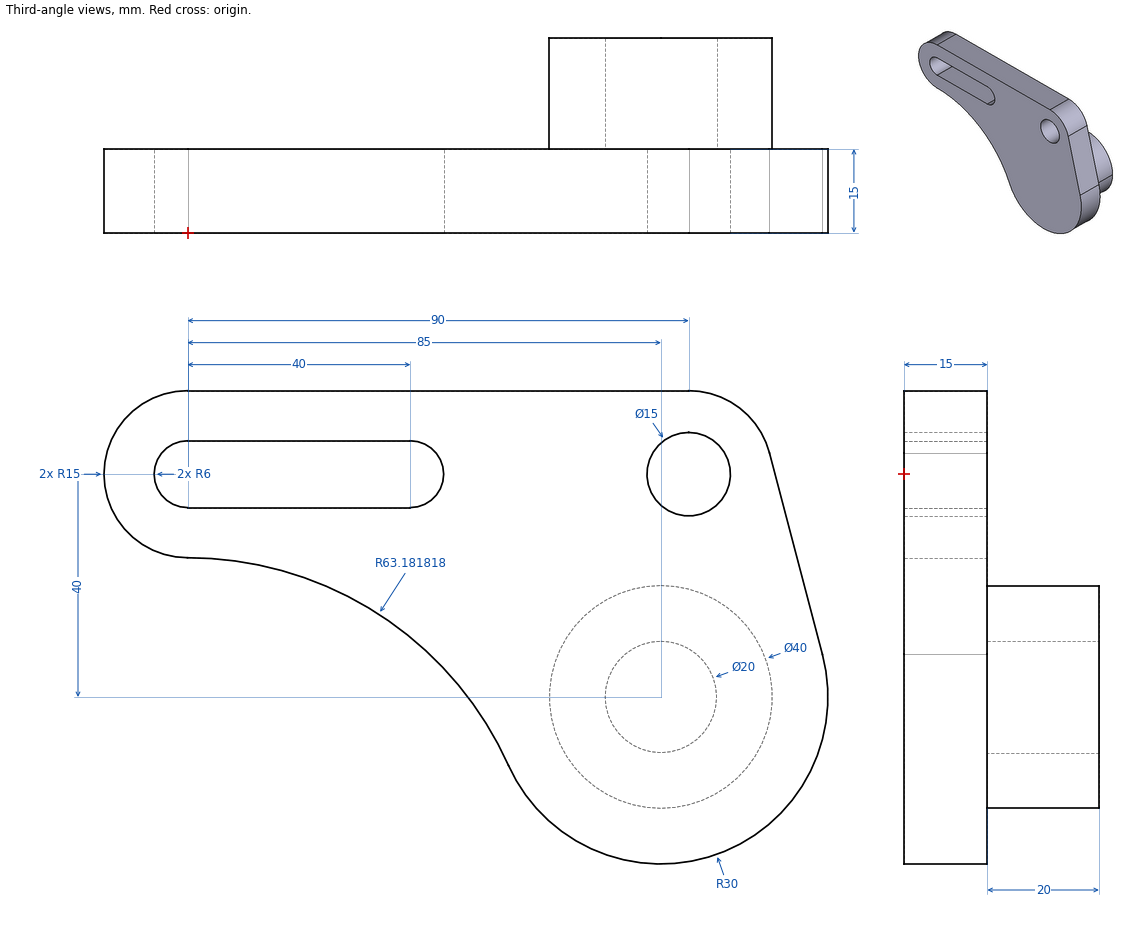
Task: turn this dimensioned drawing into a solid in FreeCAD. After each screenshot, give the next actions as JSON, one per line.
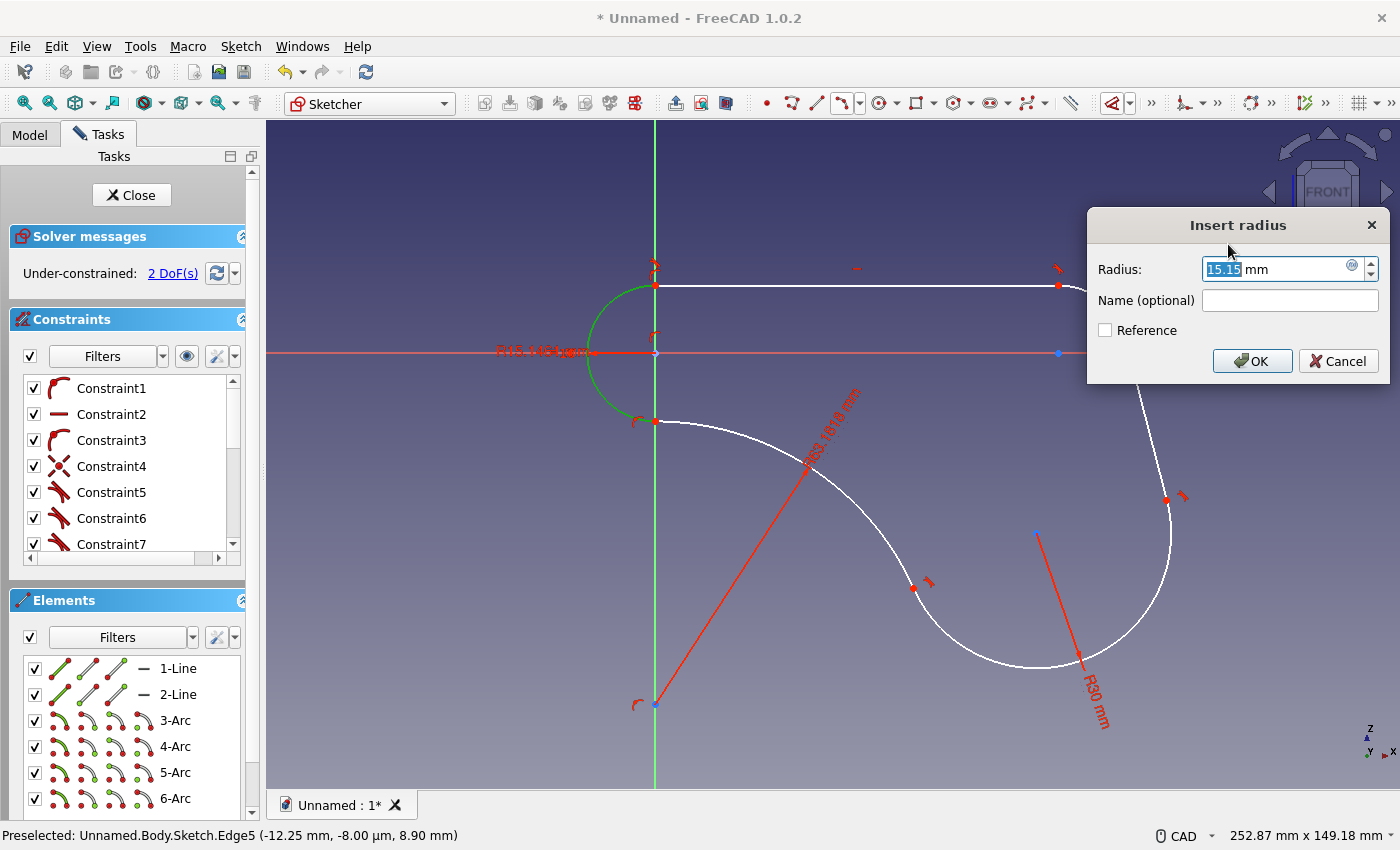
{"action": "type", "text": "15"}
{"action": "key", "text": "Return"}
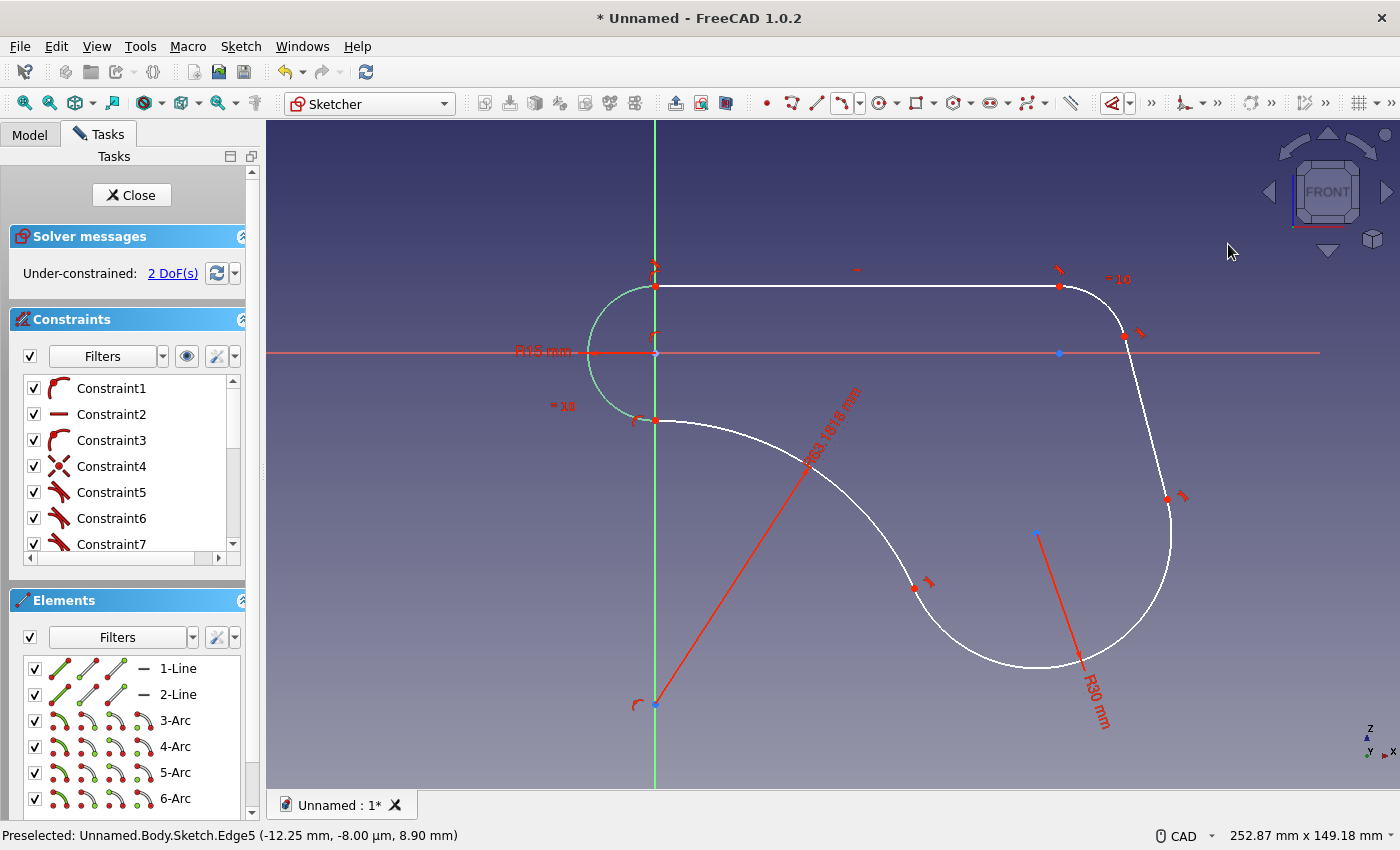
{"action": "left_click", "coordinate": [777, 286]}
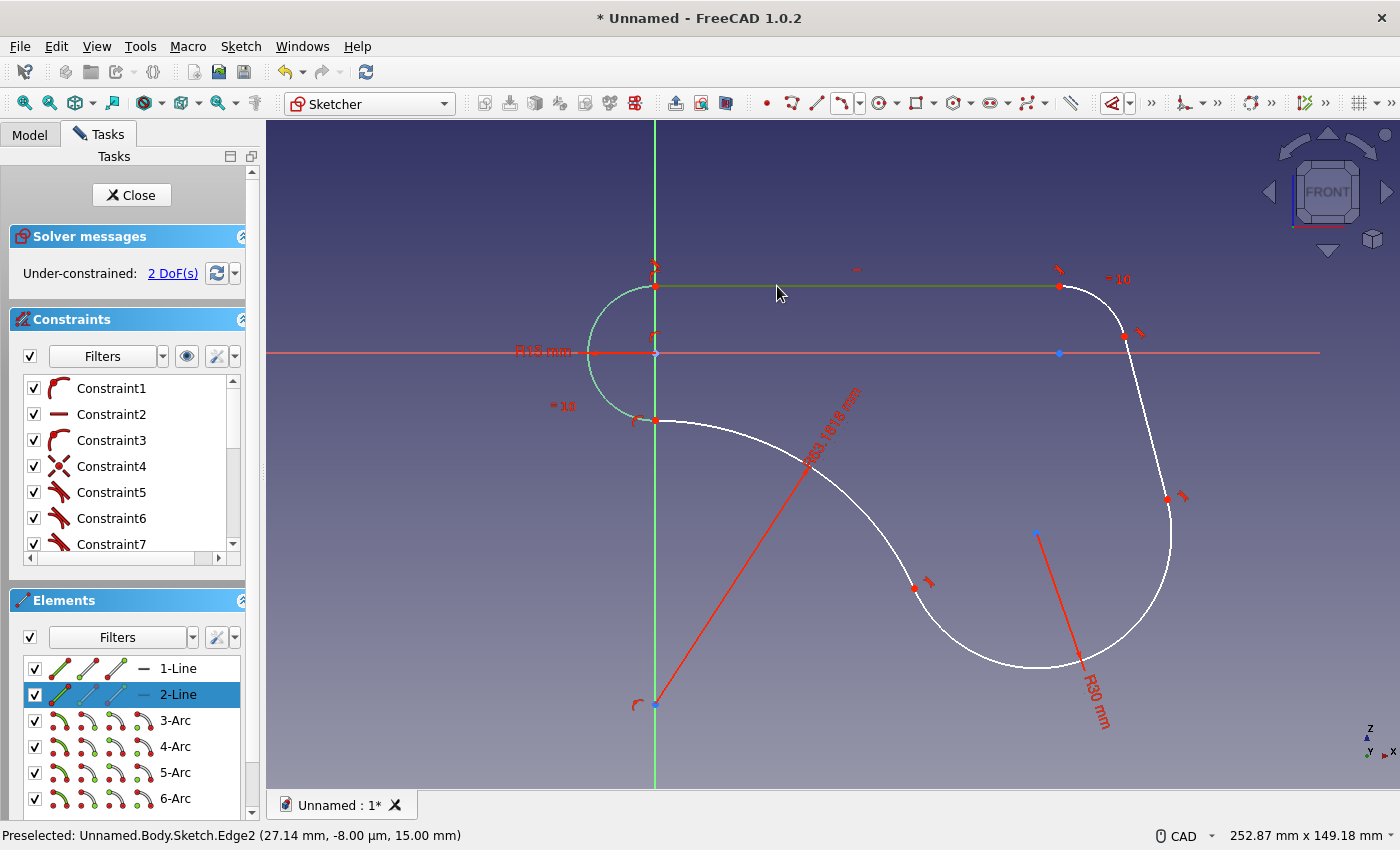
{"action": "left_click", "coordinate": [1130, 104]}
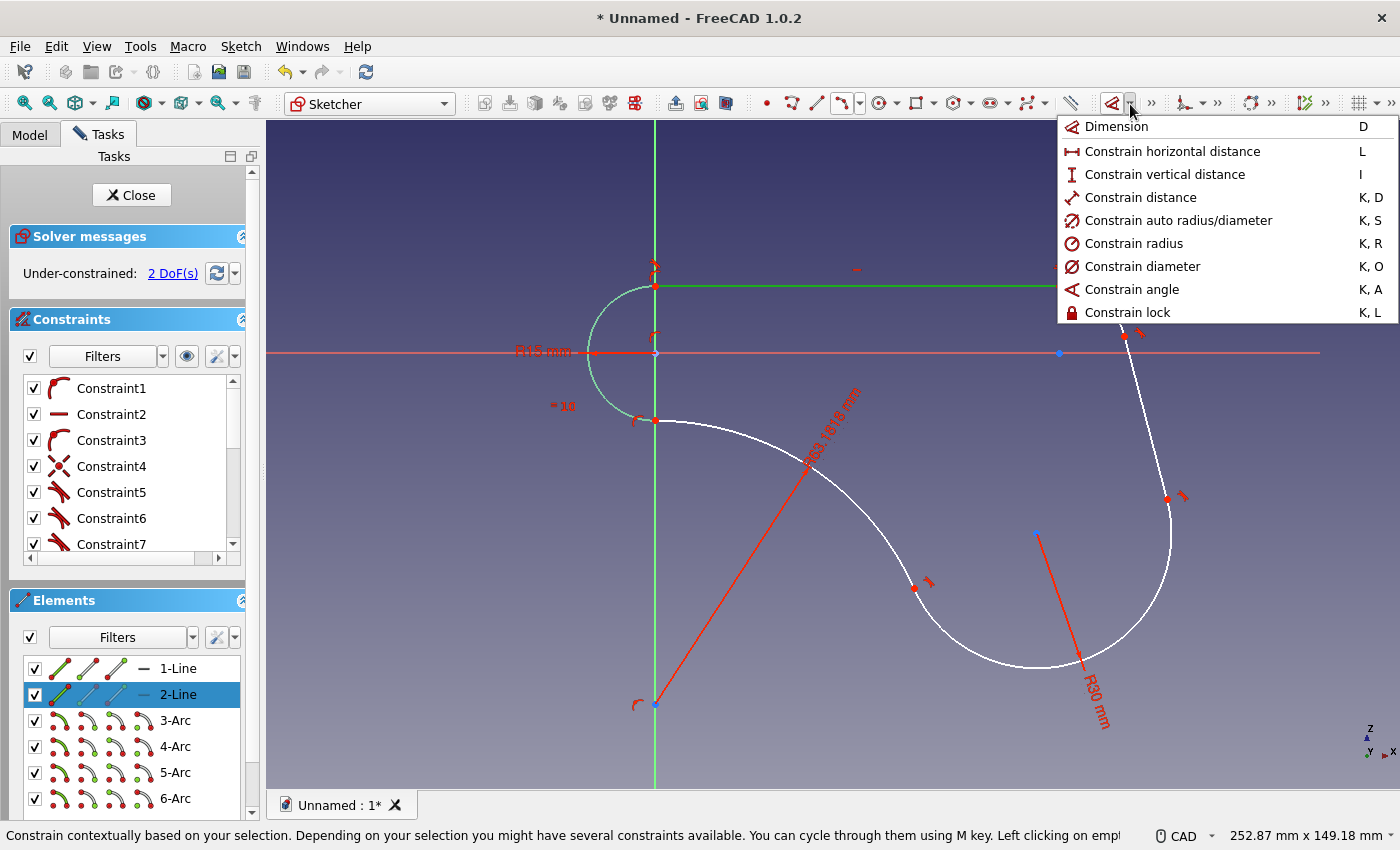
{"action": "left_click", "coordinate": [1228, 152]}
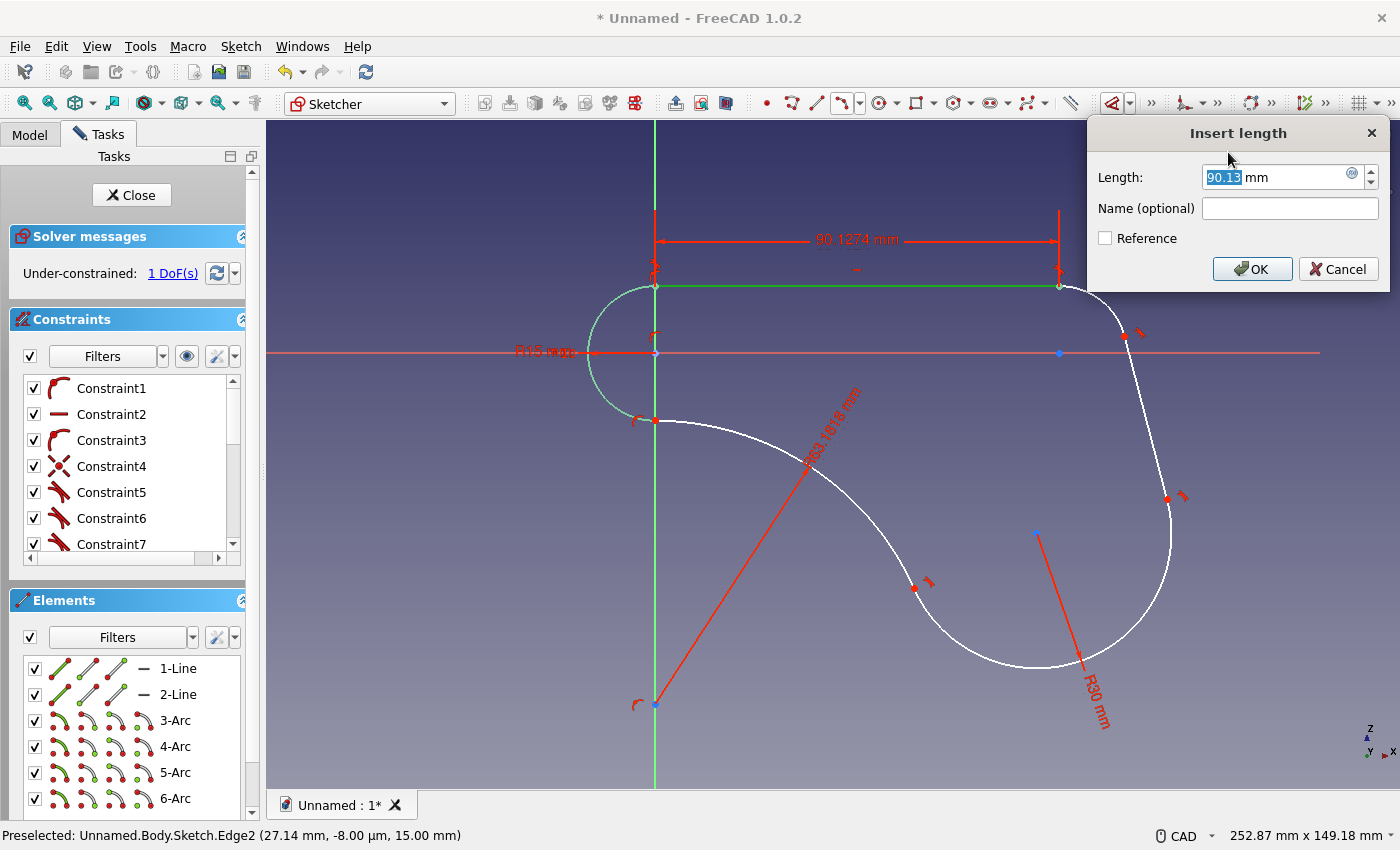
{"action": "type", "text": "90"}
{"action": "key", "text": "Return"}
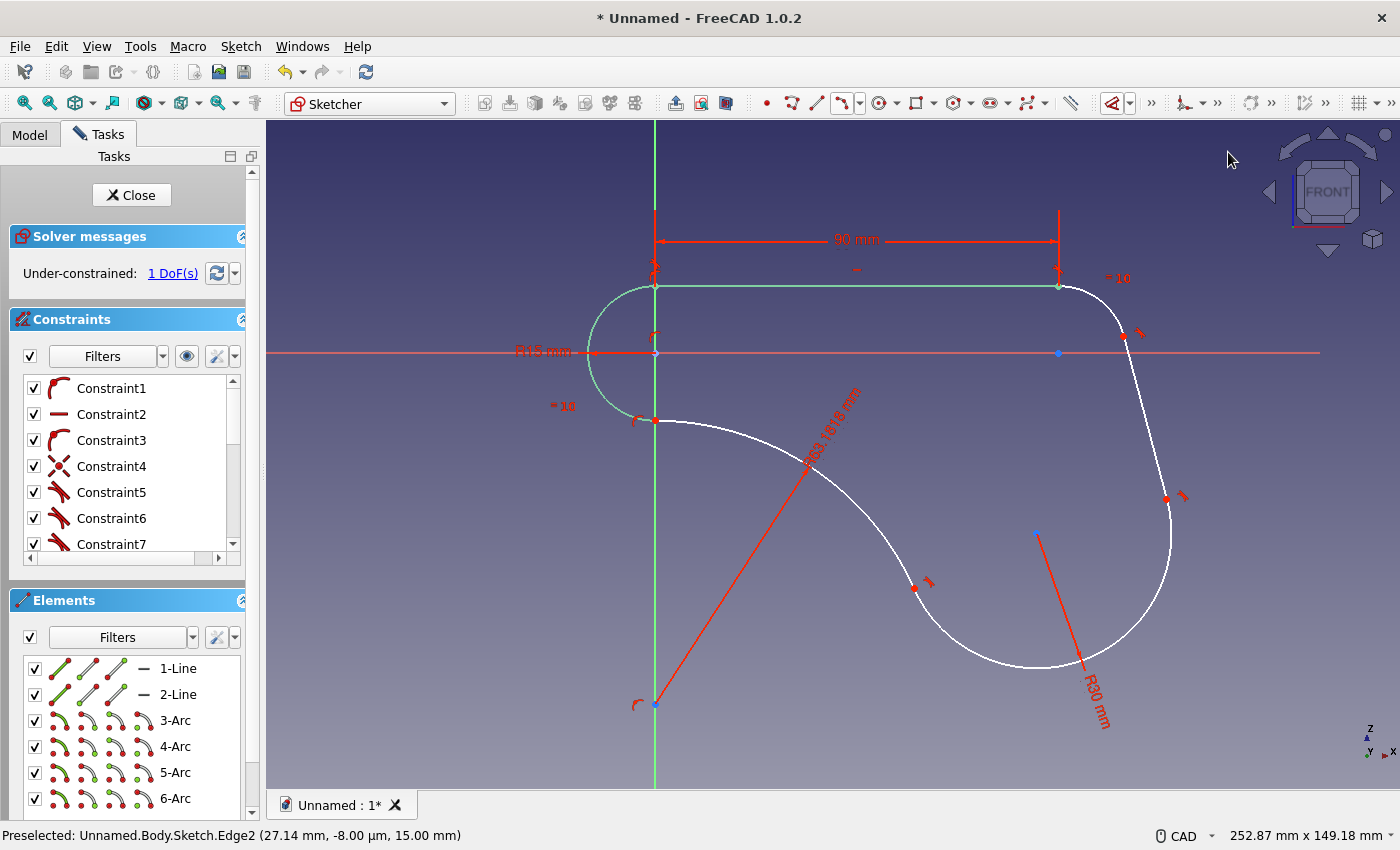
{"action": "left_click", "coordinate": [1037, 534]}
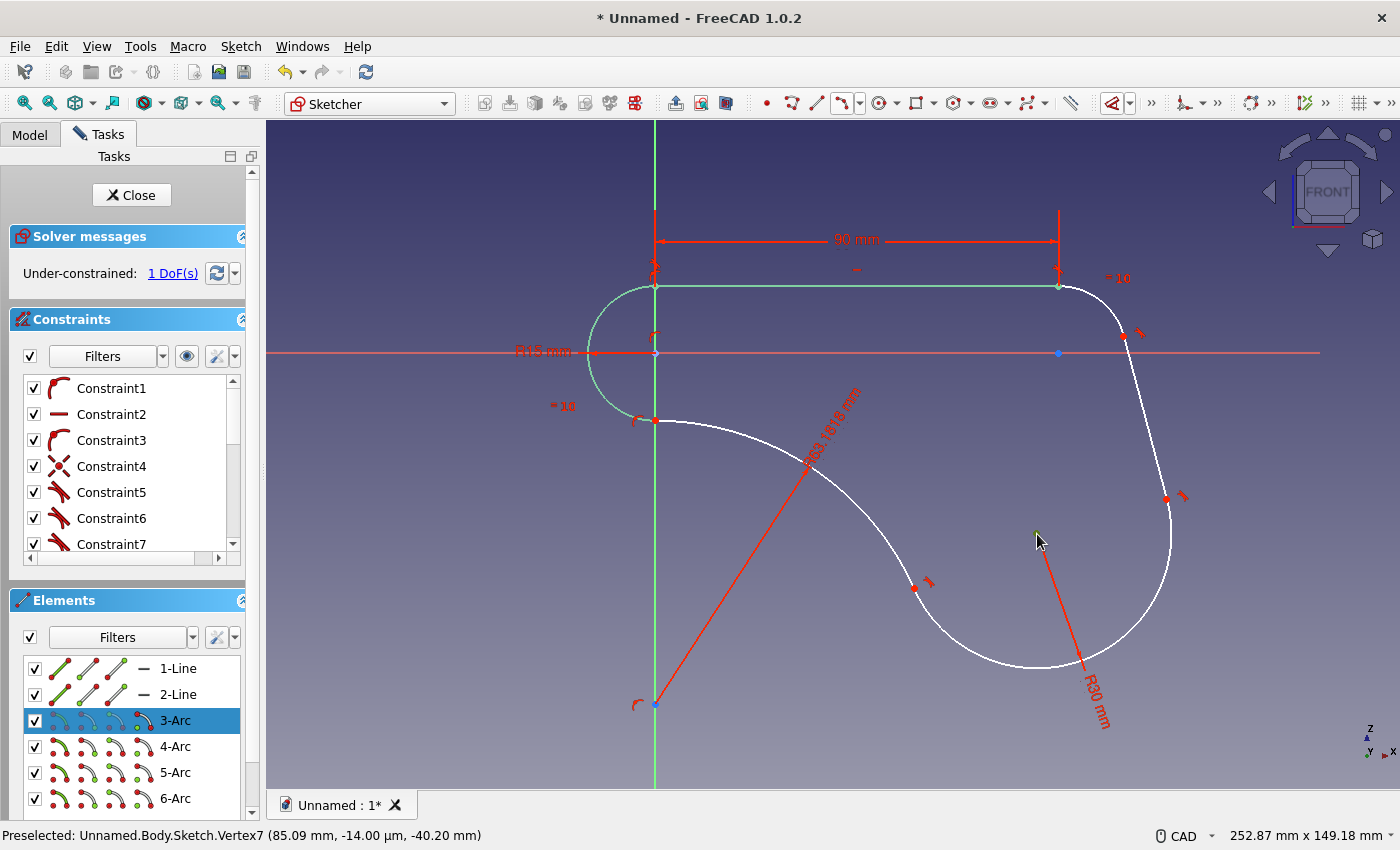
{"action": "key", "text": "l"}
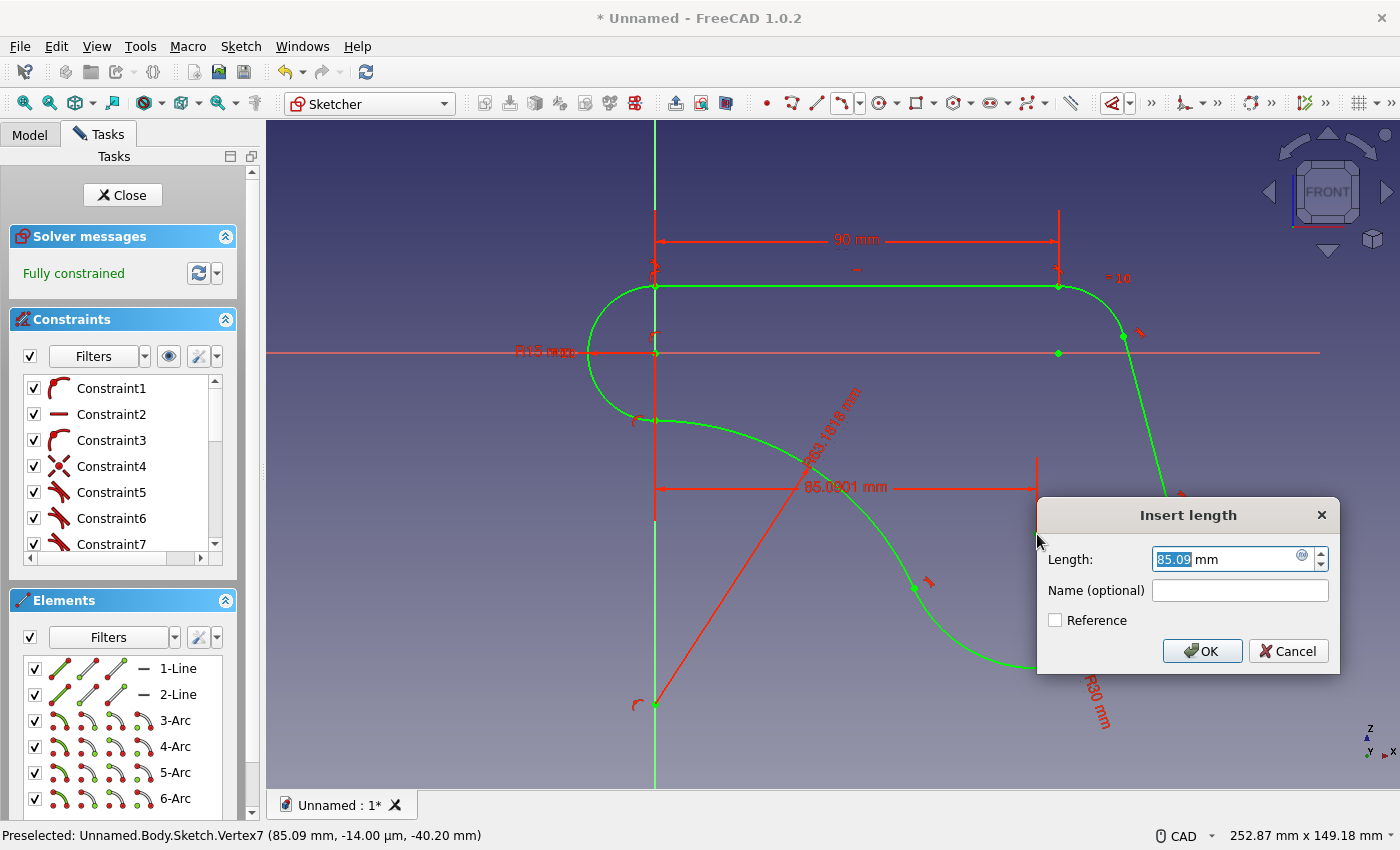
{"action": "type", "text": "85"}
{"action": "key", "text": "Return"}